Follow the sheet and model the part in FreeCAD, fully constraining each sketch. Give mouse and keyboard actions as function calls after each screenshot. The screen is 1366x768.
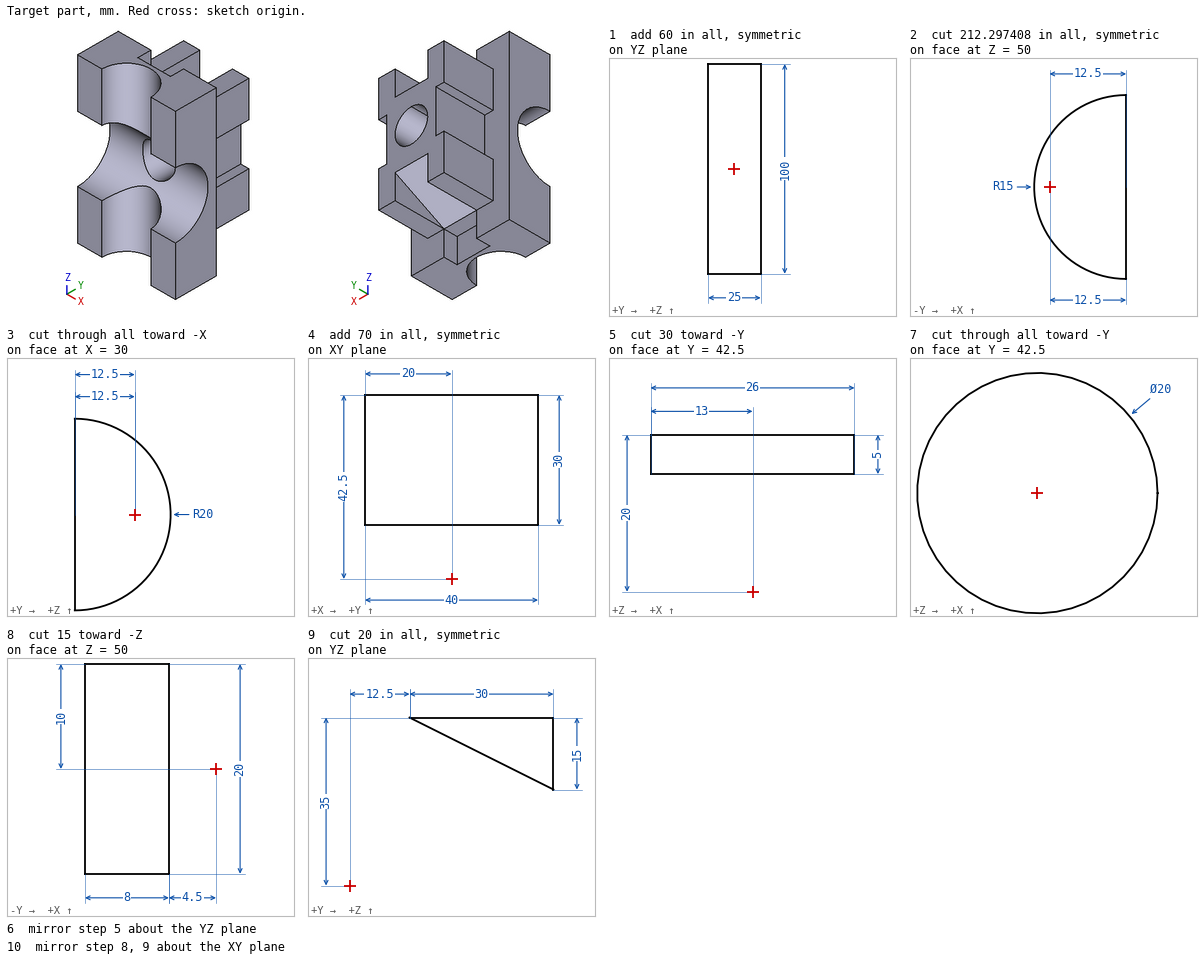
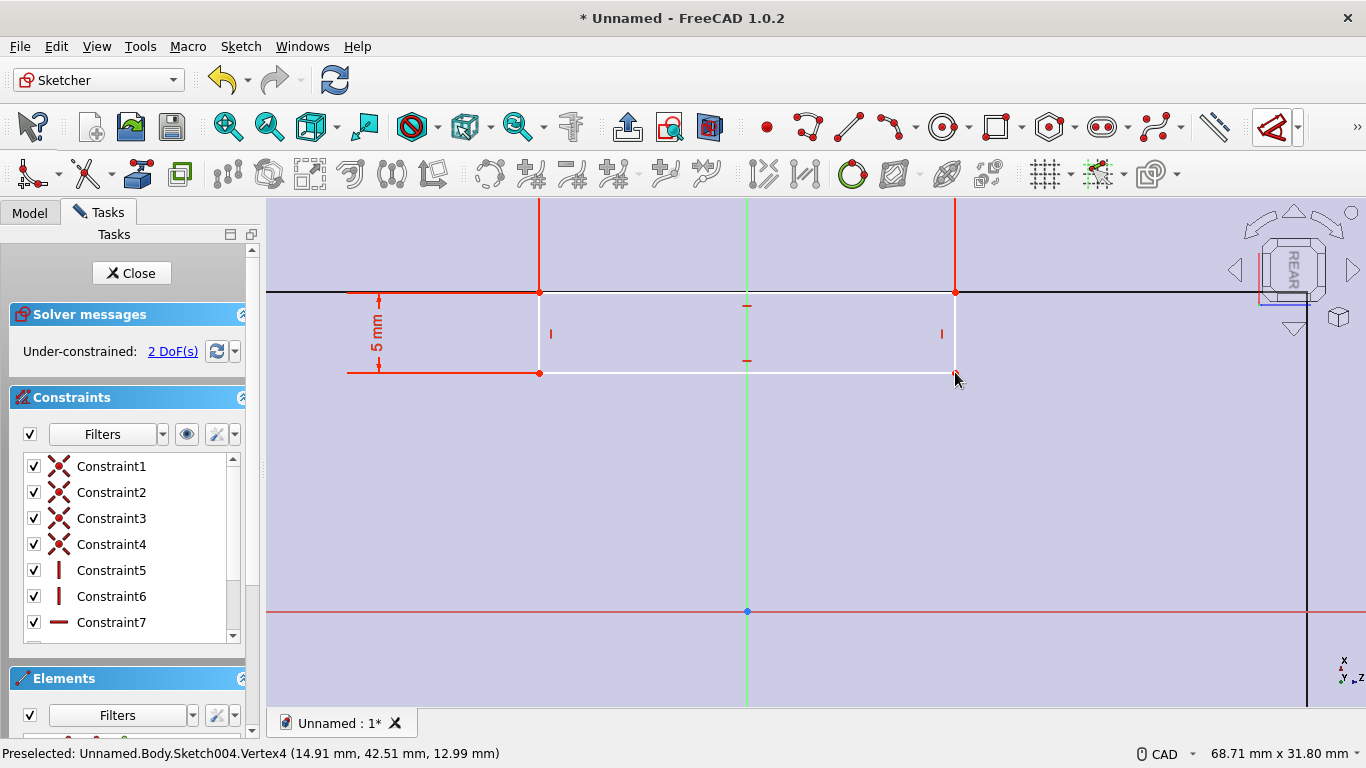
click(539, 293)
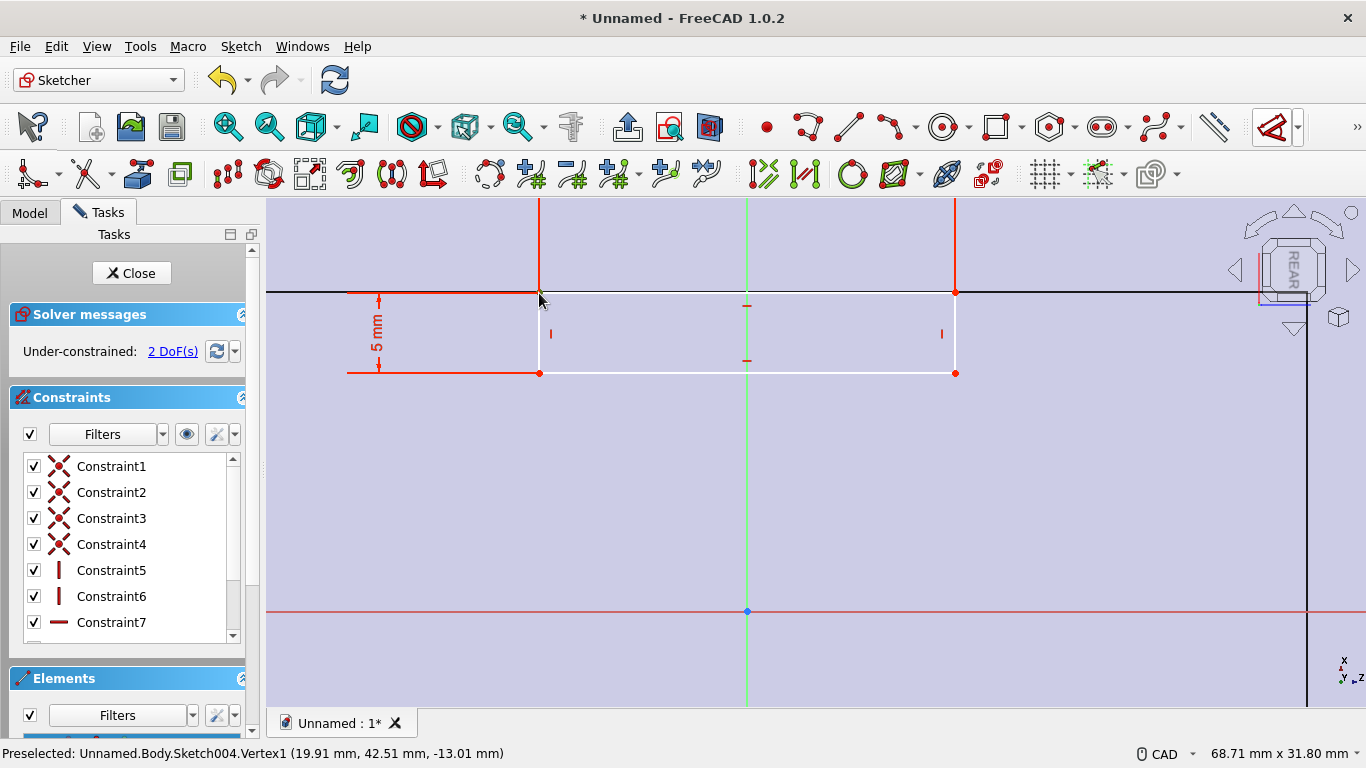
key(l)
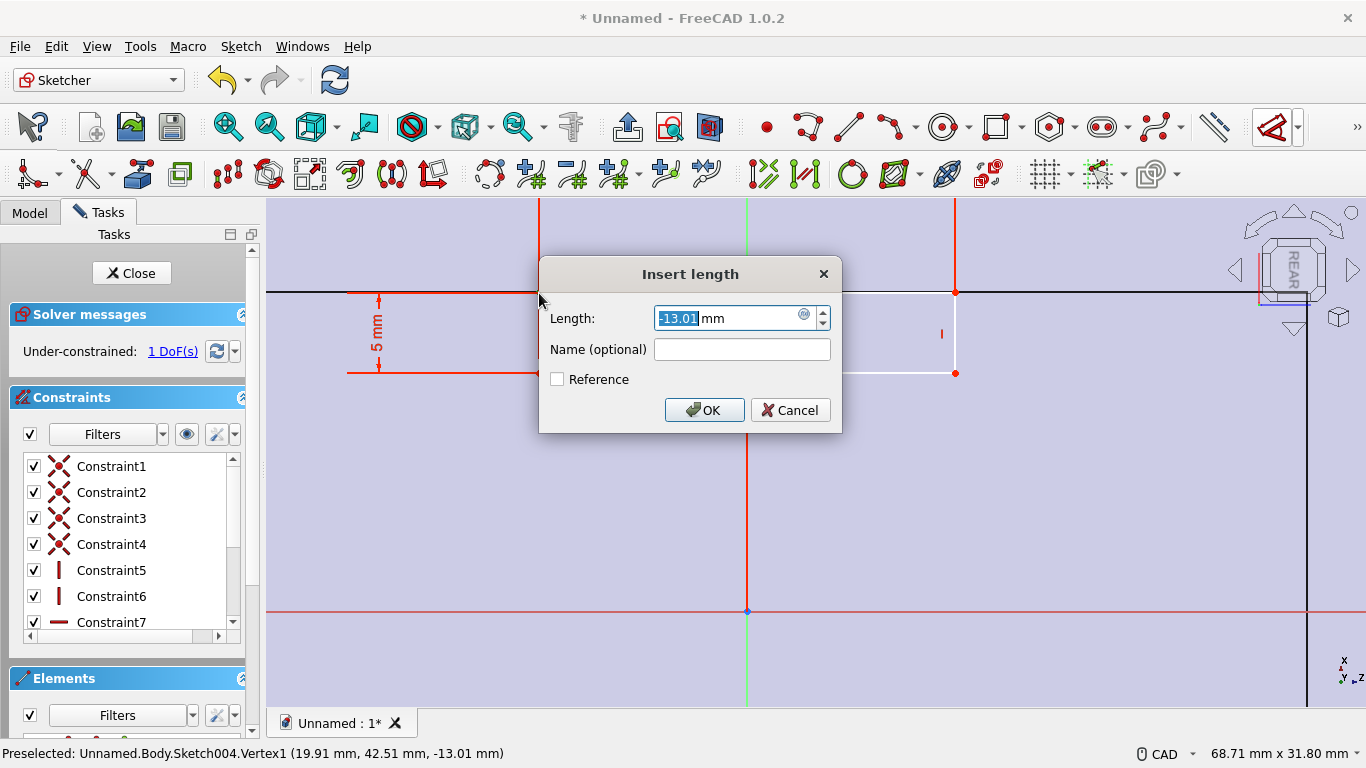
text(-13)
key(Return)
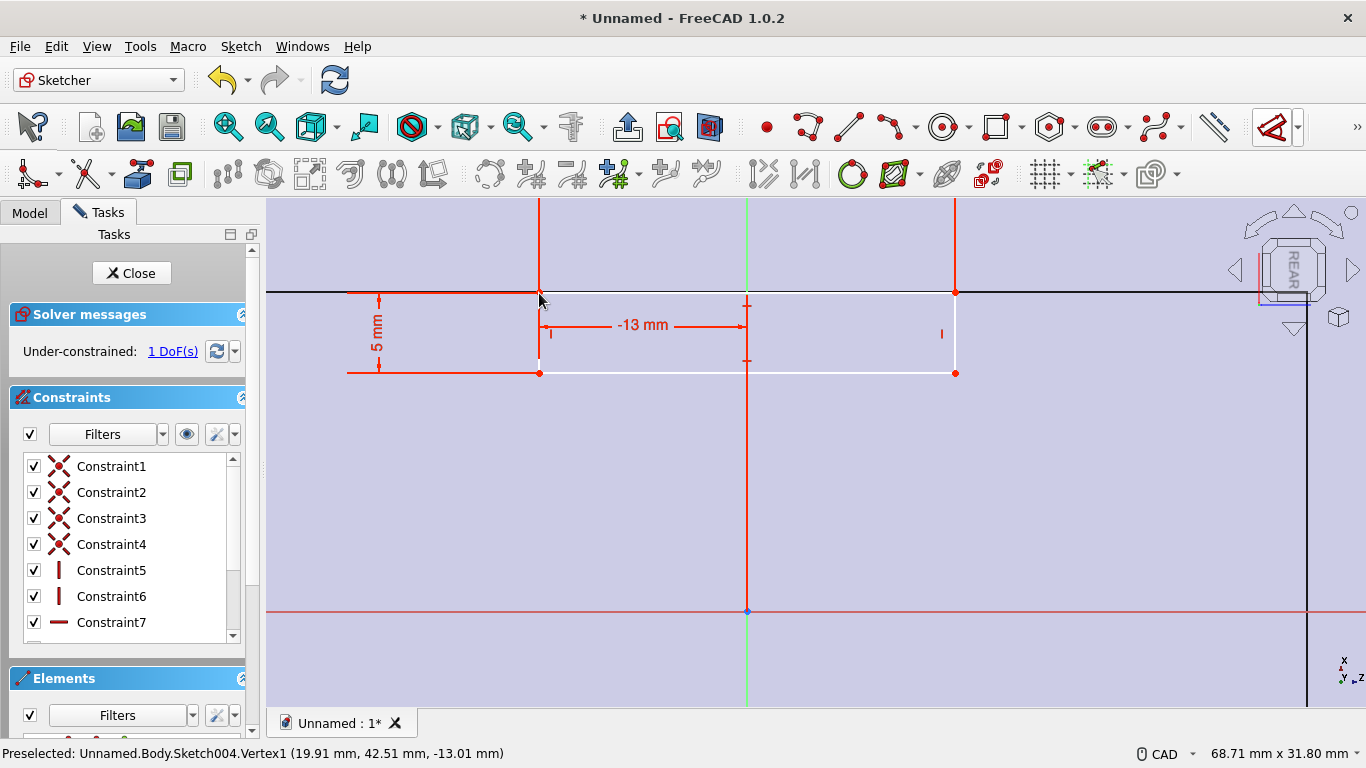
click(539, 293)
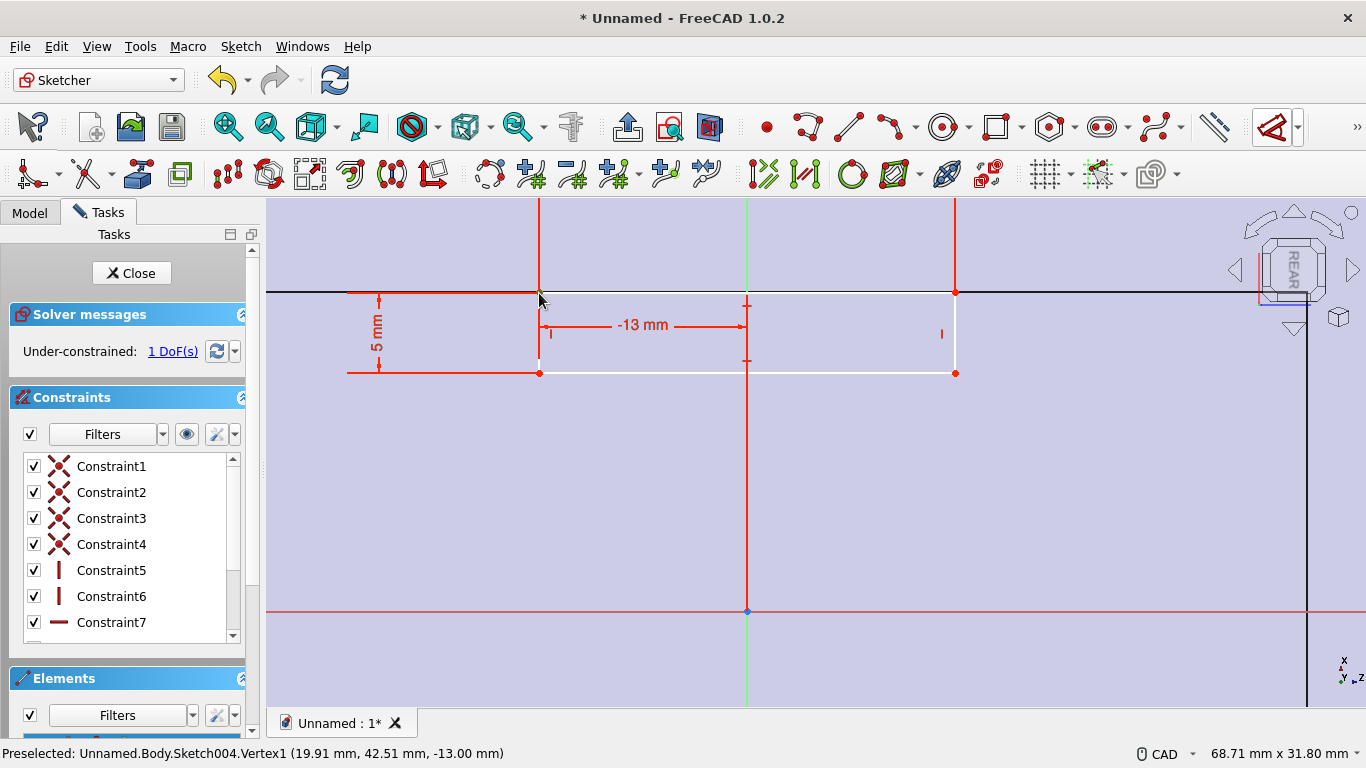
key(i)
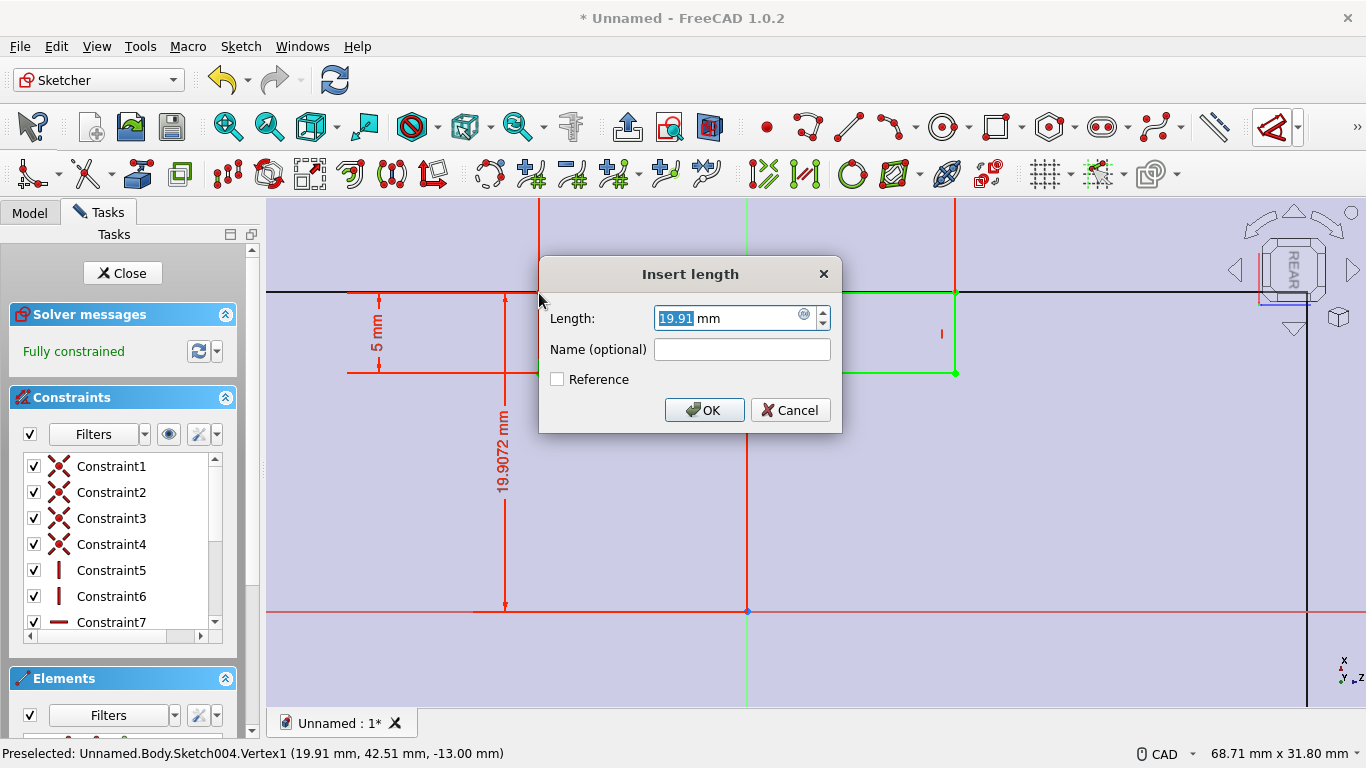
text(20)
key(Return)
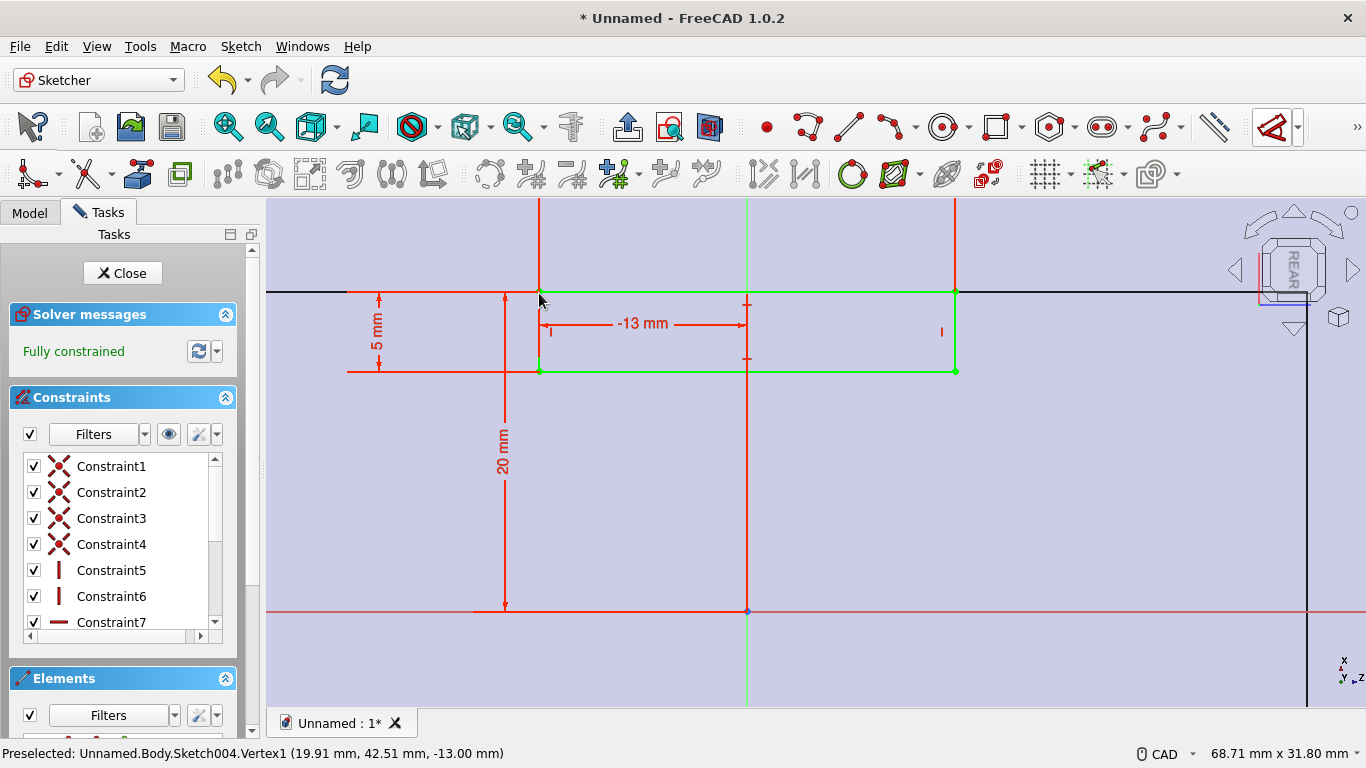
click(123, 273)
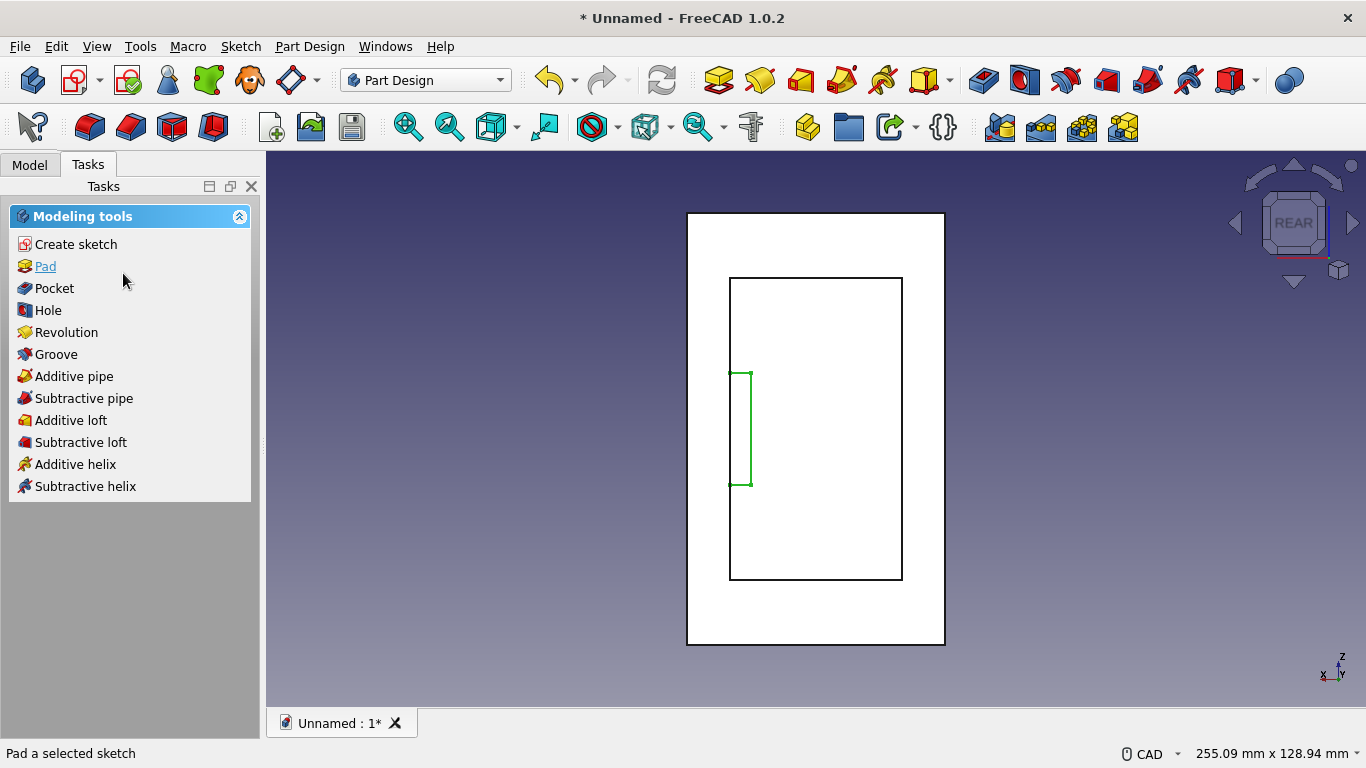
click(984, 80)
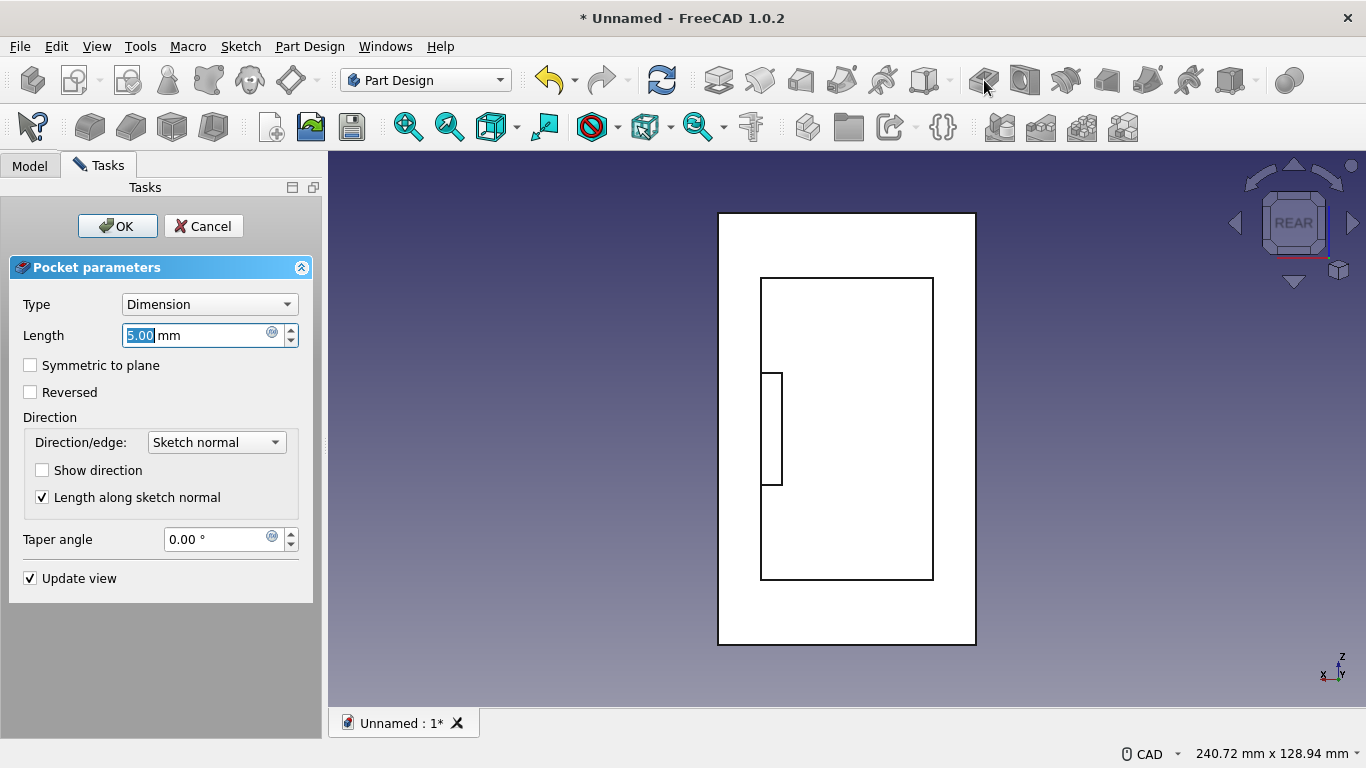
text(30)
key(Tab)